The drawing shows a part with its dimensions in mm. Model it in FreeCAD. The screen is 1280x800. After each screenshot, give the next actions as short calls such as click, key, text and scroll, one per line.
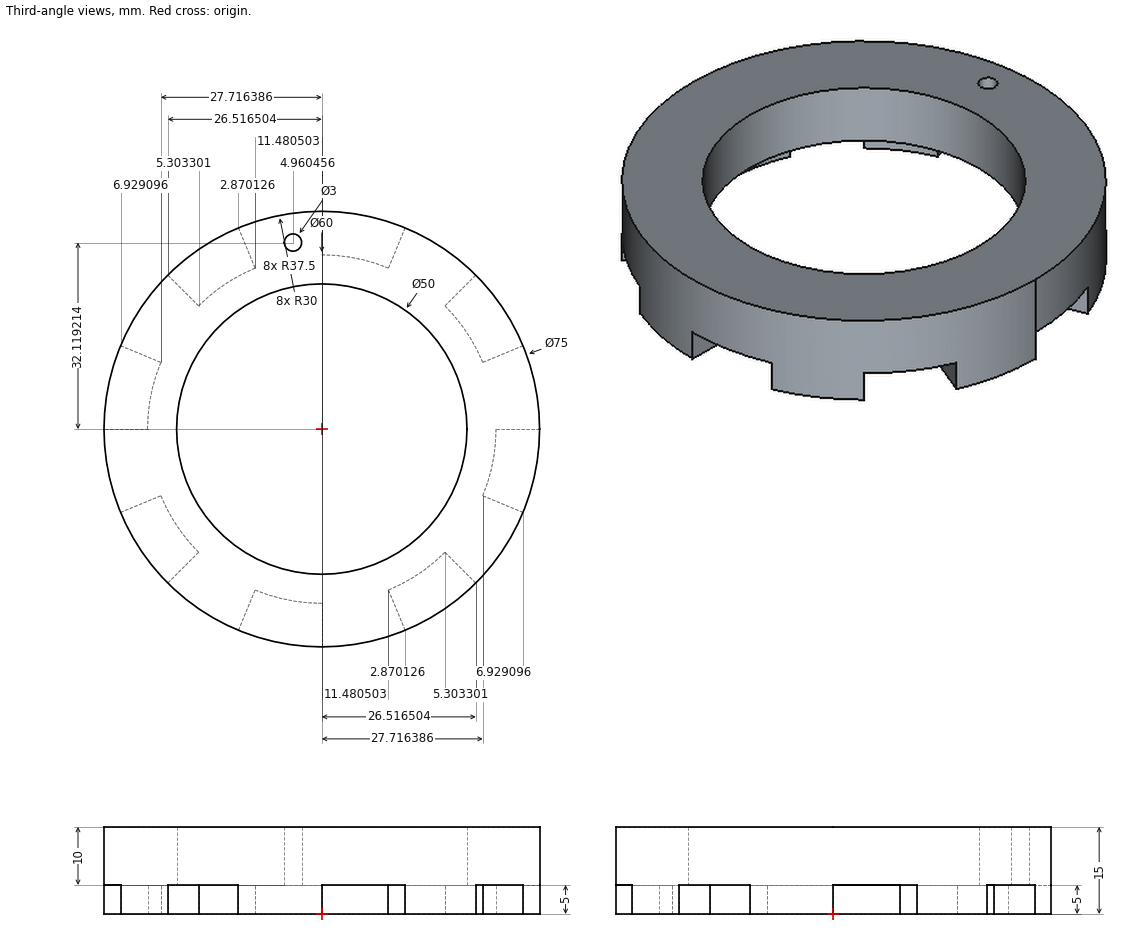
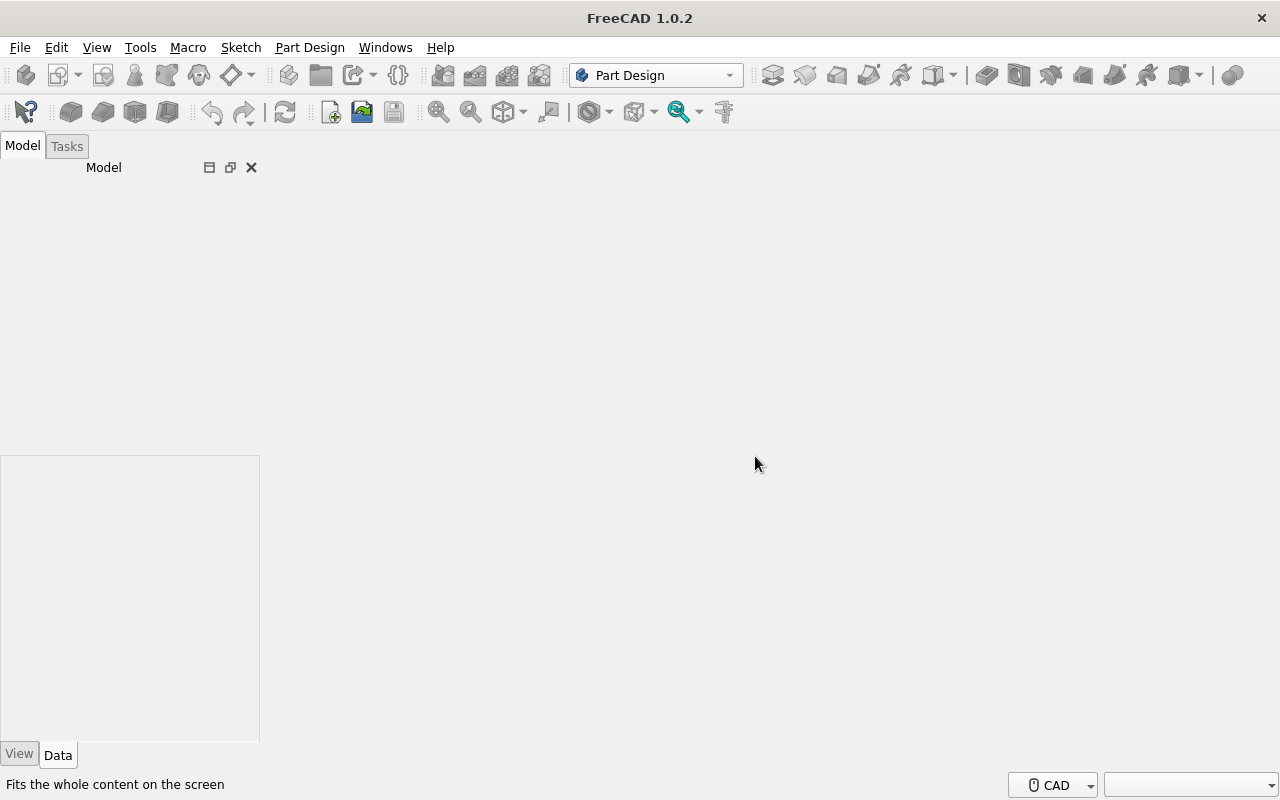
key(ctrl+n)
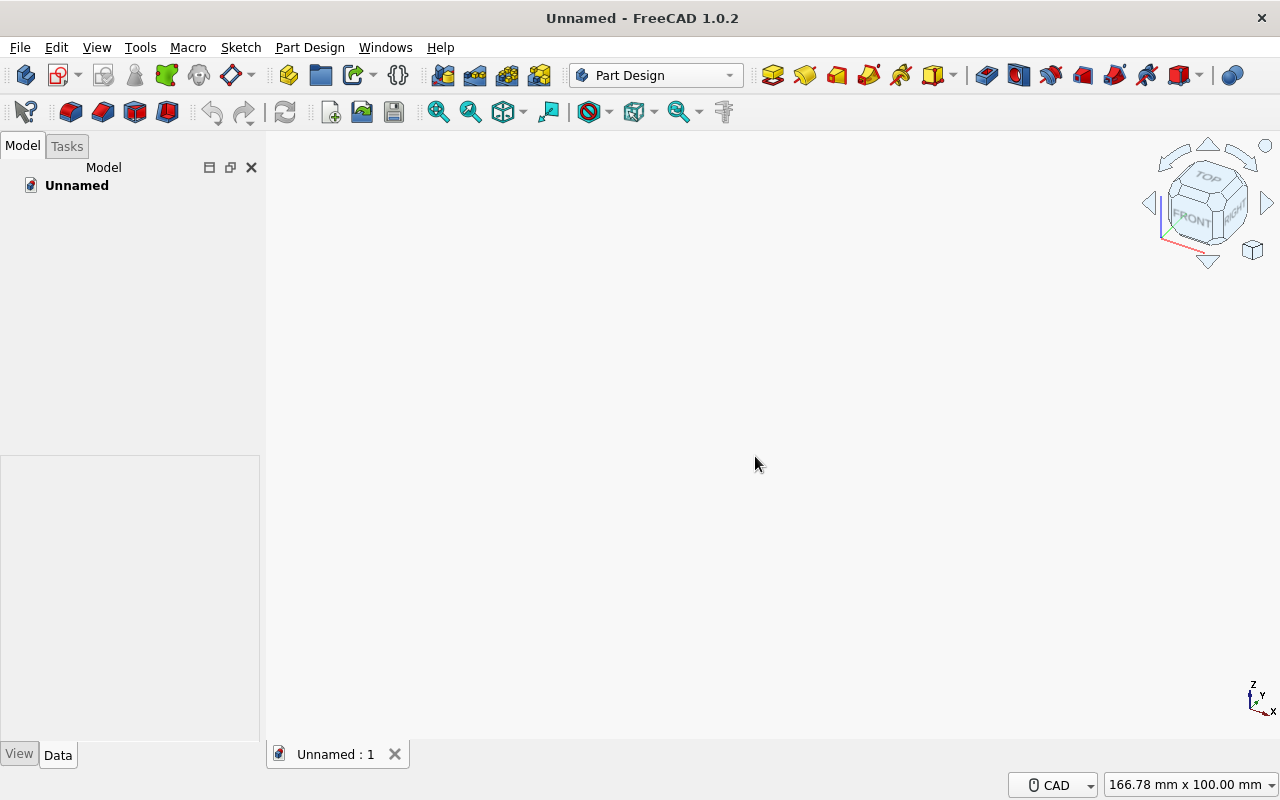
click(58, 76)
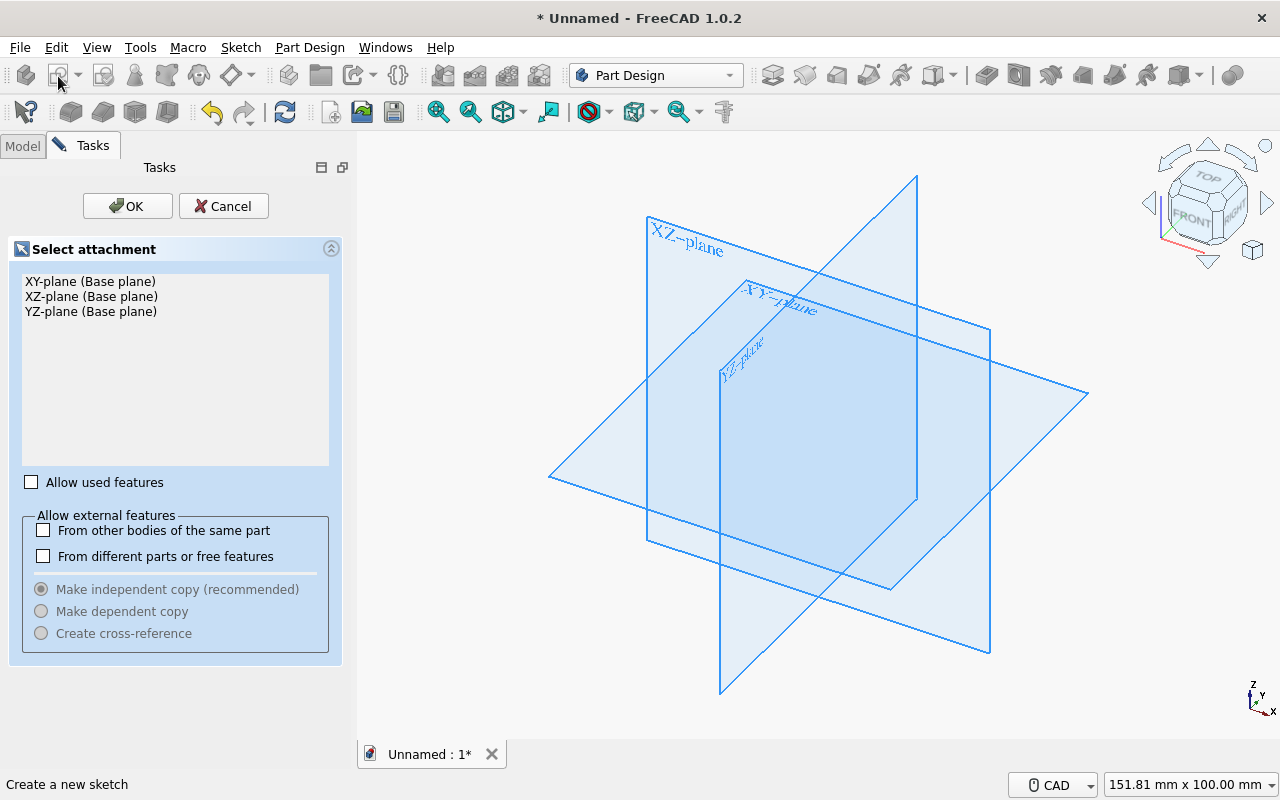
click(82, 282)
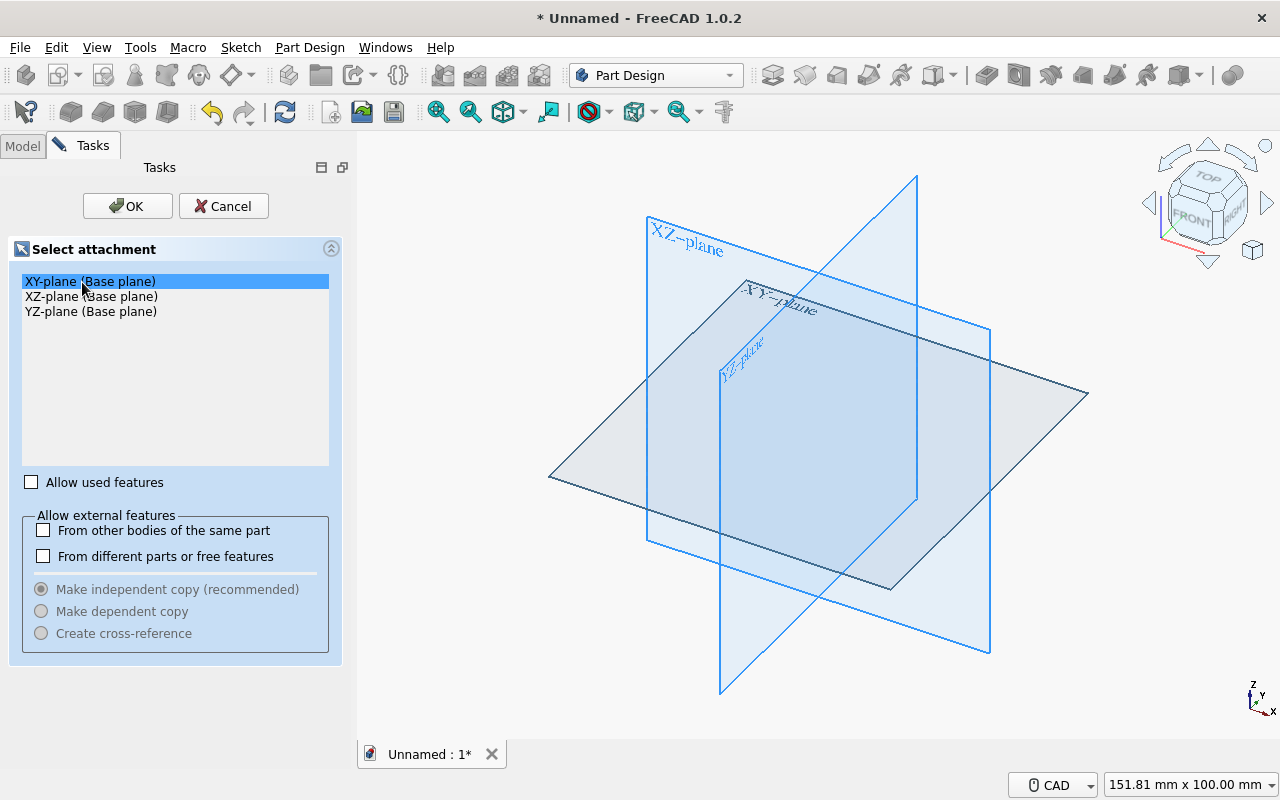
click(128, 206)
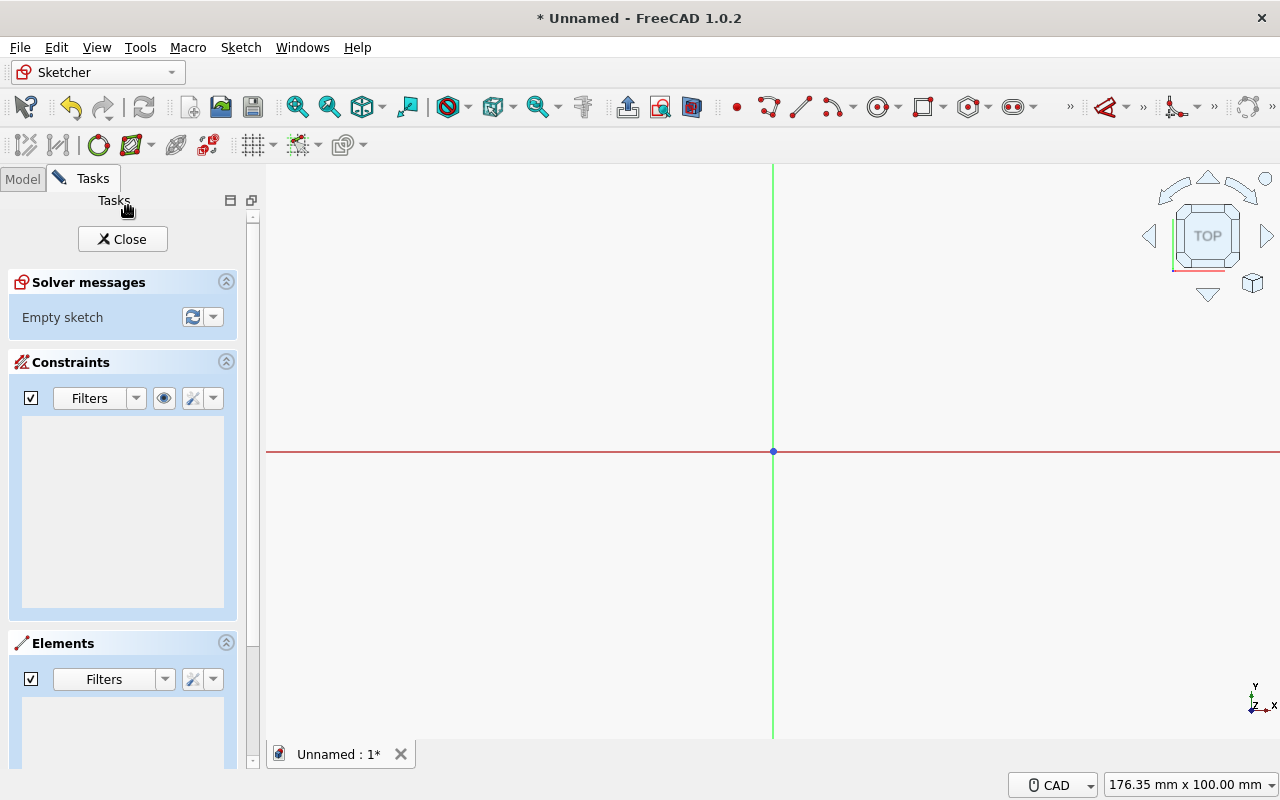
key(g)
key(c)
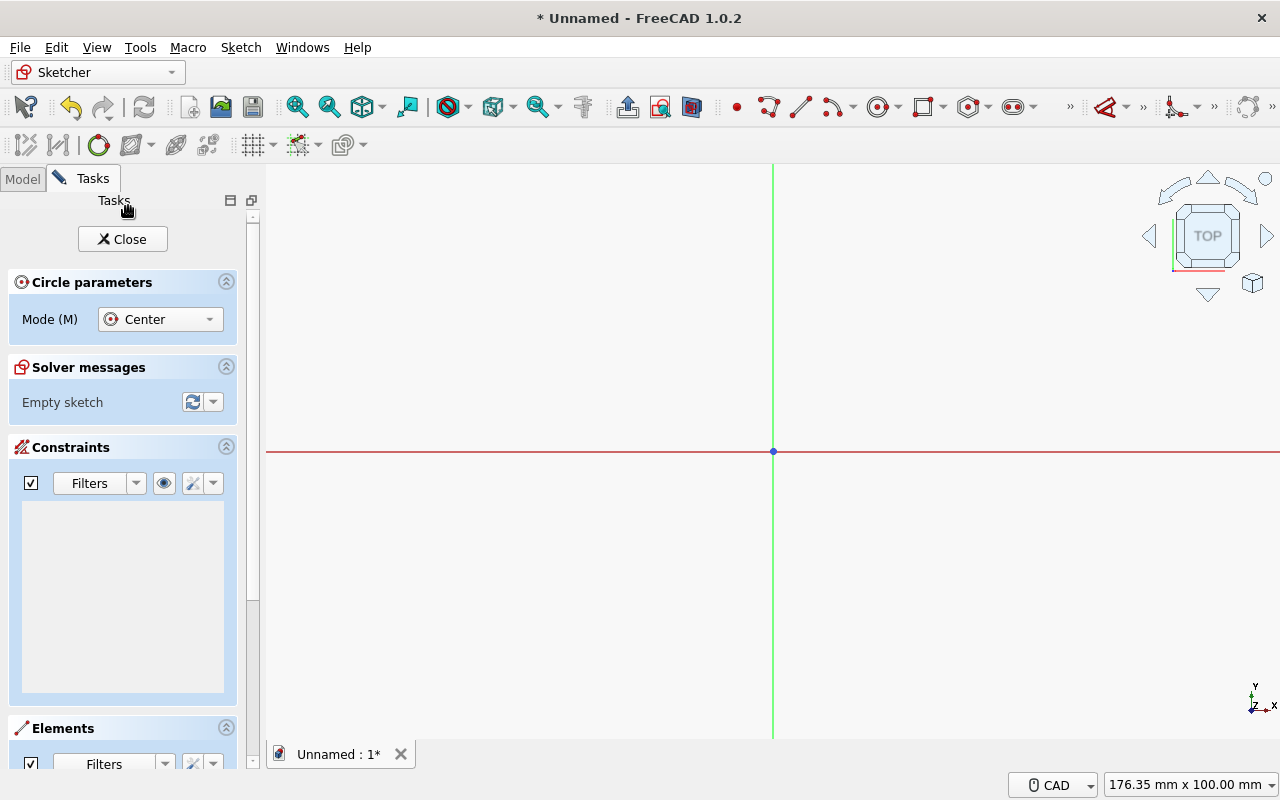
click(773, 452)
move(925, 299)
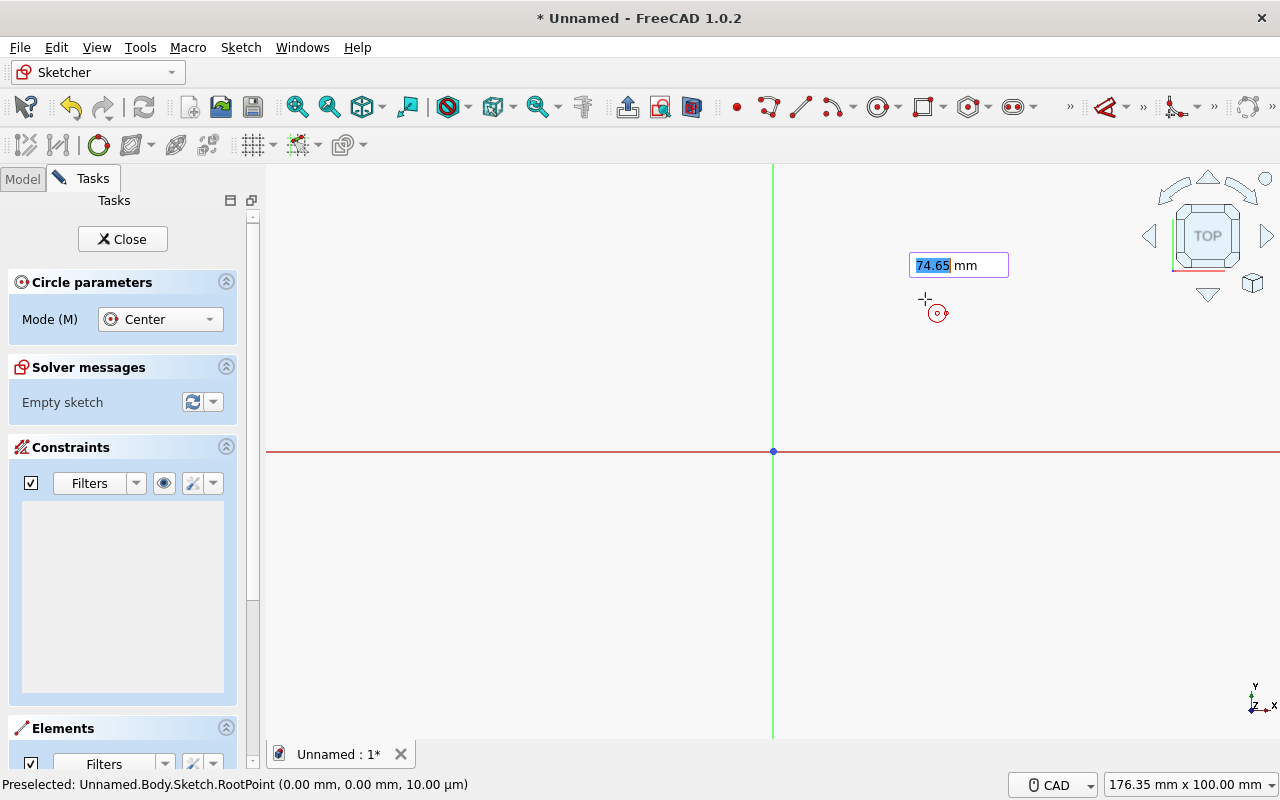
text(75)
key(Return)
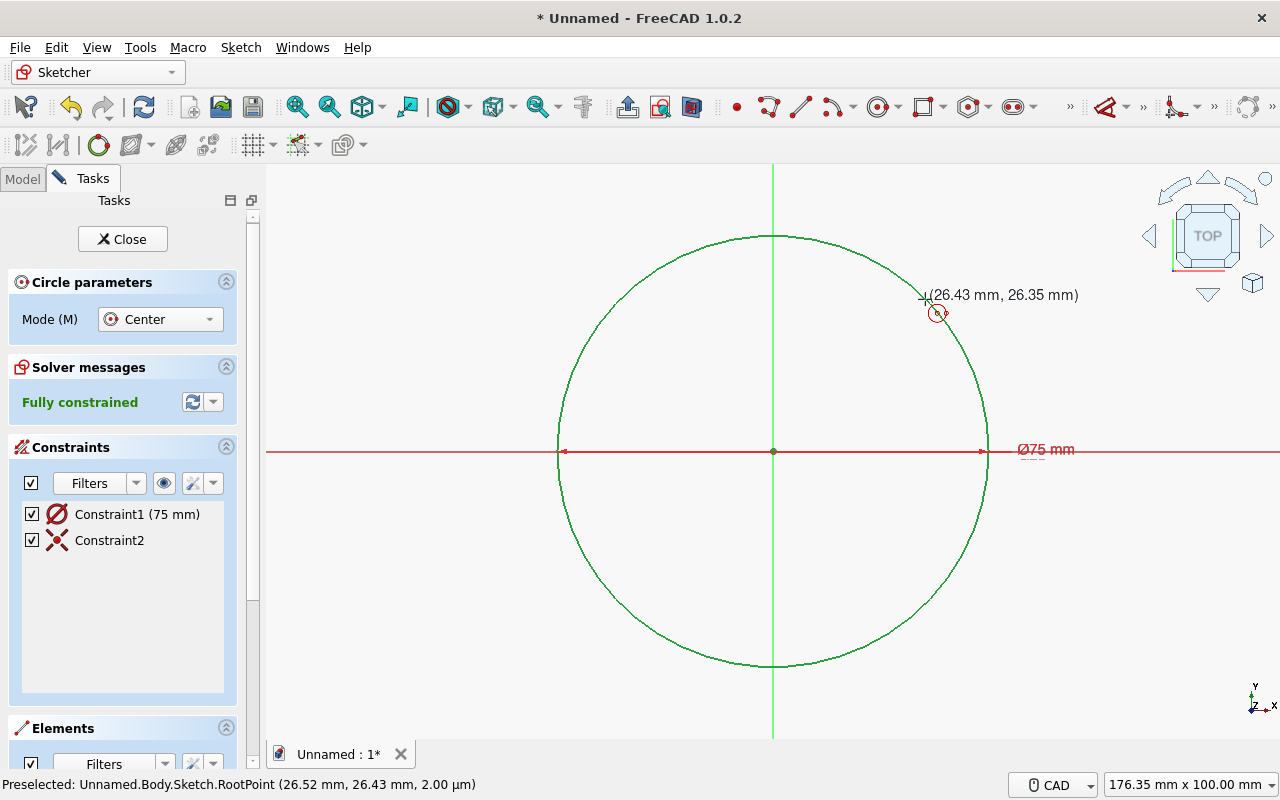
click(773, 452)
move(875, 350)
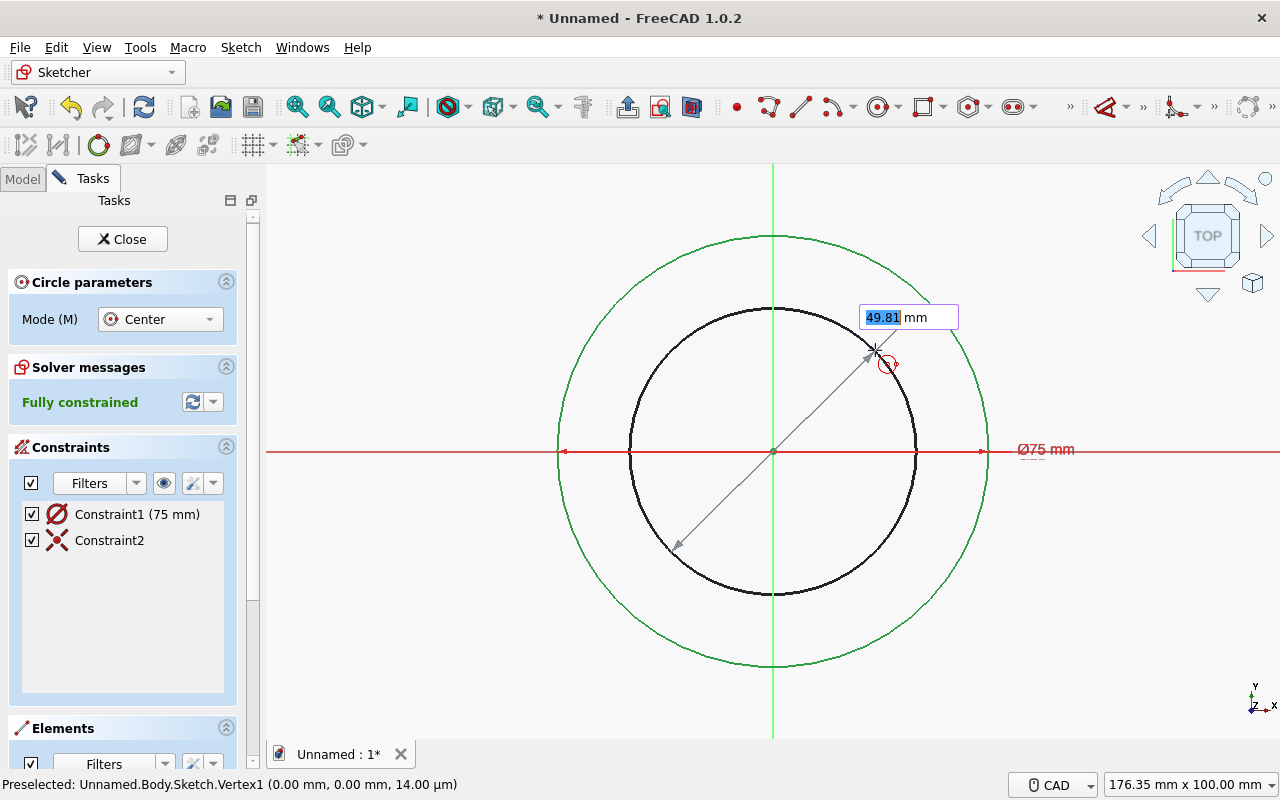
text(50)
key(Return)
key(Escape)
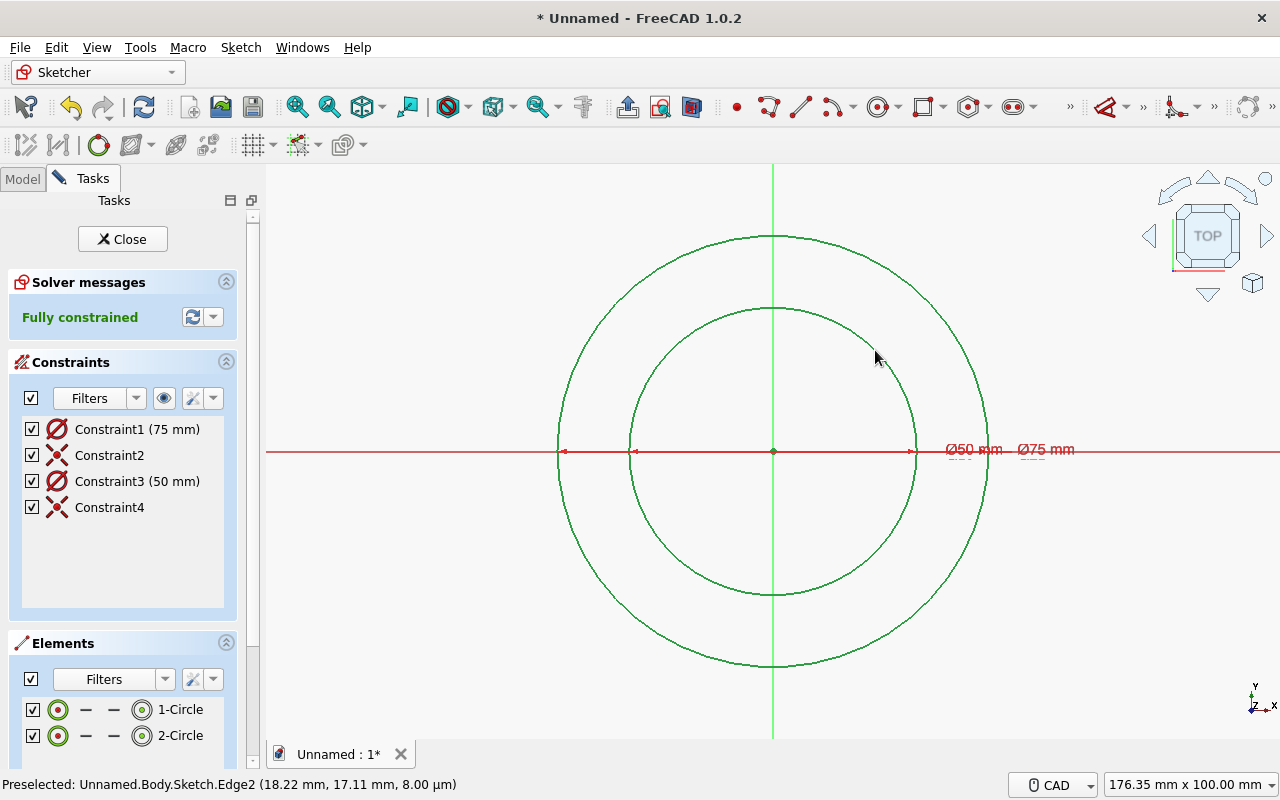
click(123, 239)